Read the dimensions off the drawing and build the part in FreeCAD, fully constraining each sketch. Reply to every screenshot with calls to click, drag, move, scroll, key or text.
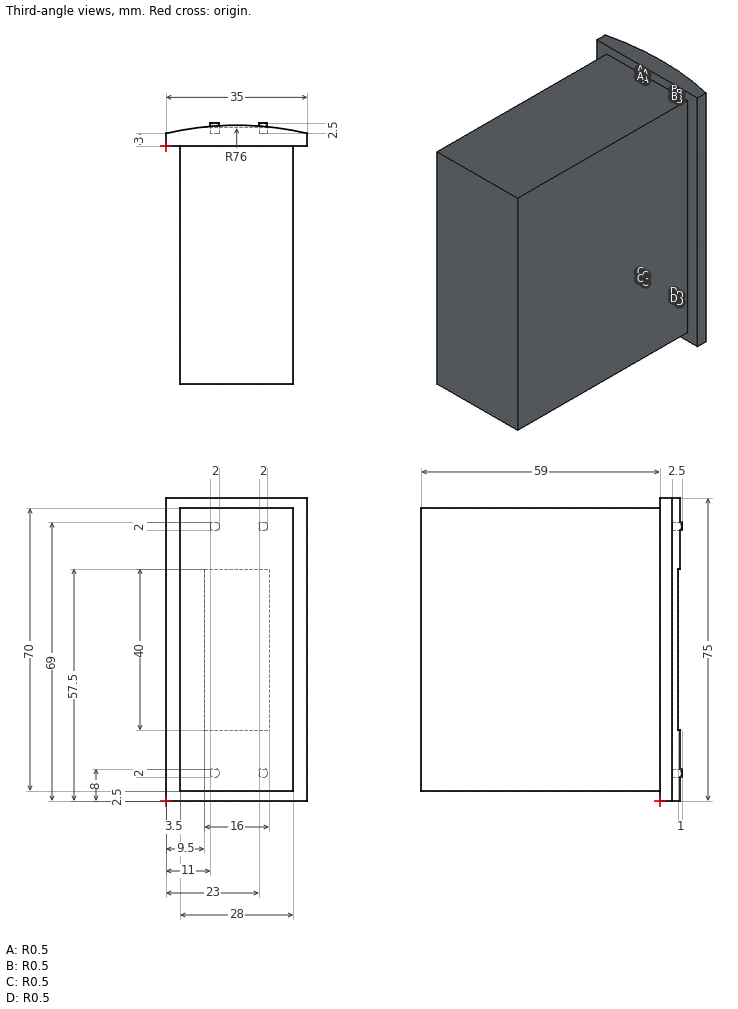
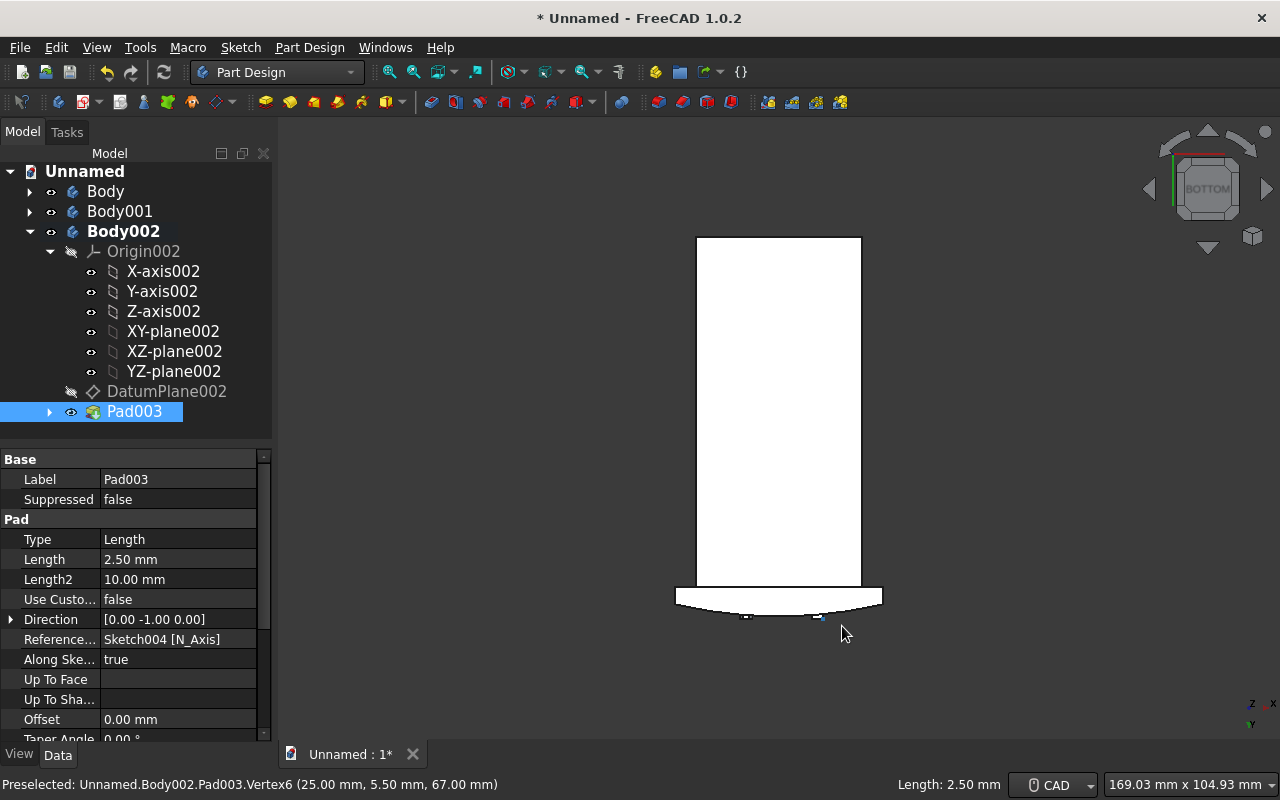
key(4)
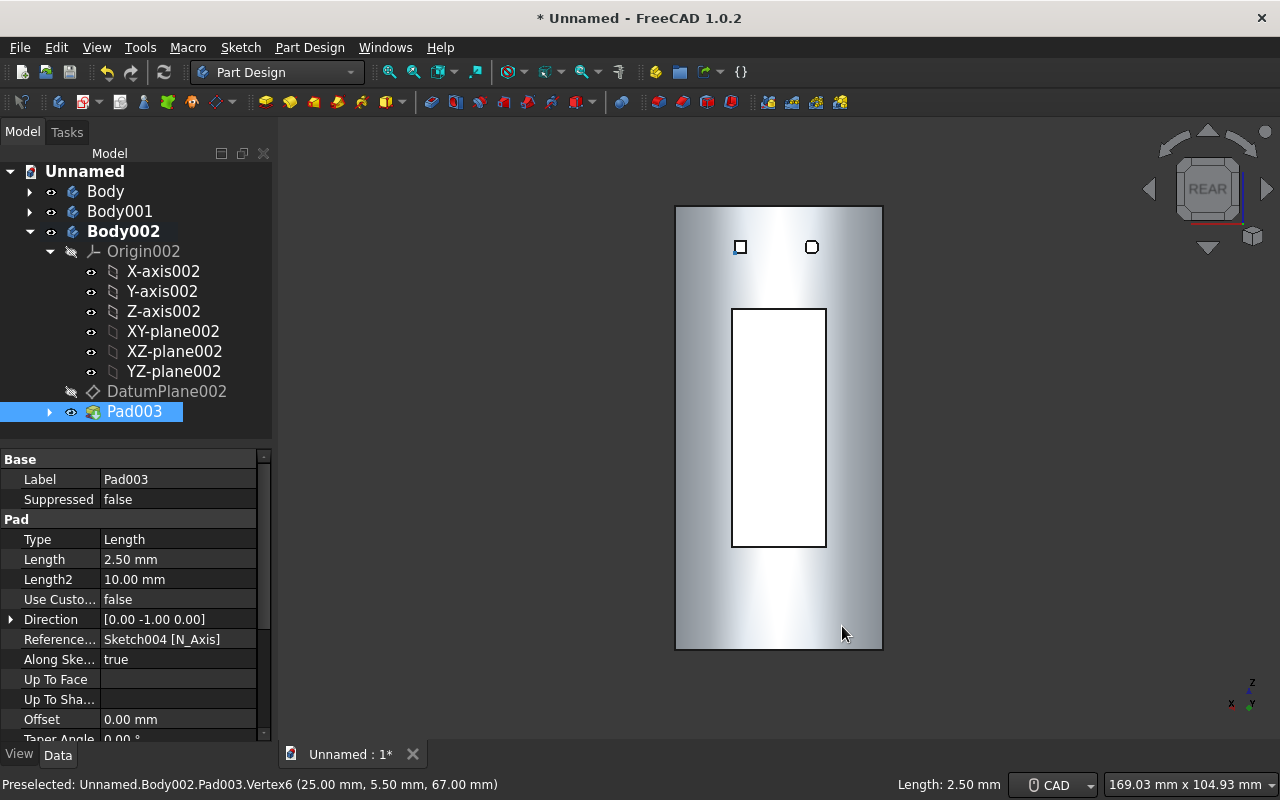
key(v)
key(f)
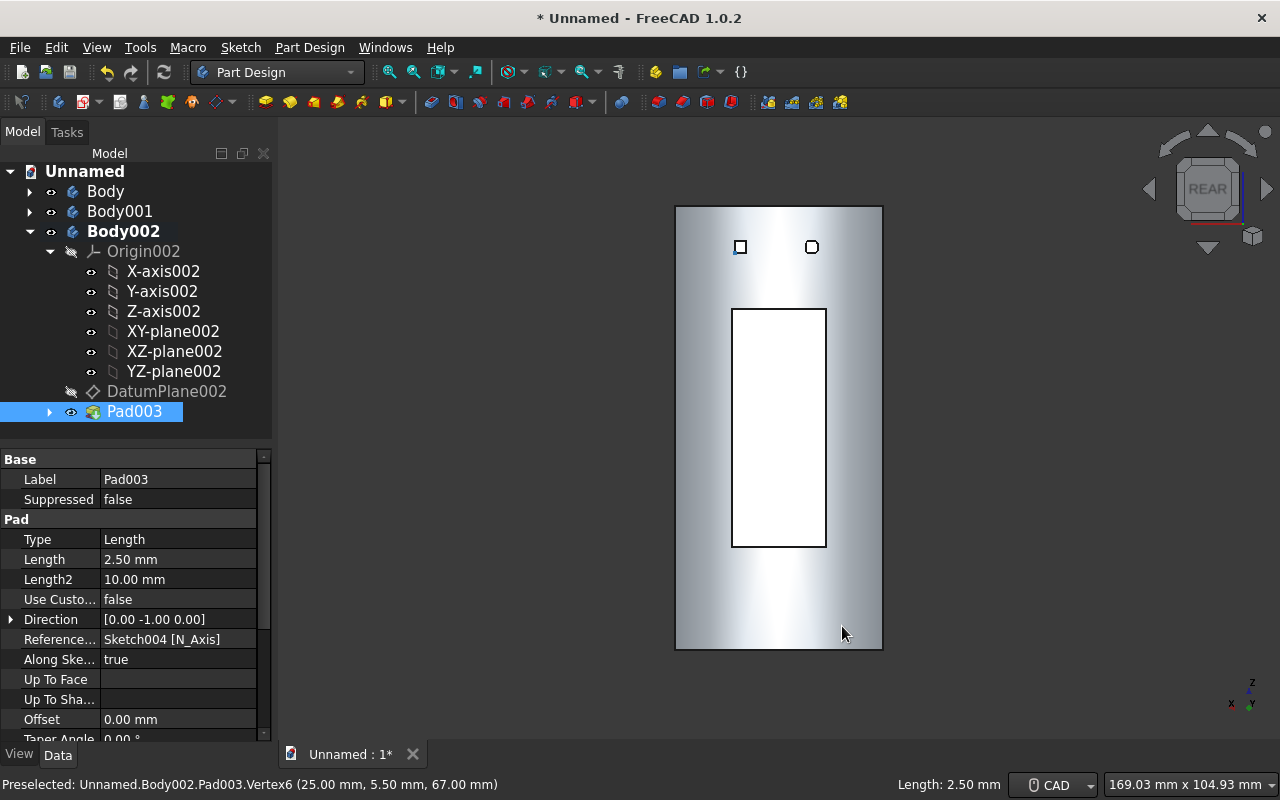
scroll(746, 240, up, 5)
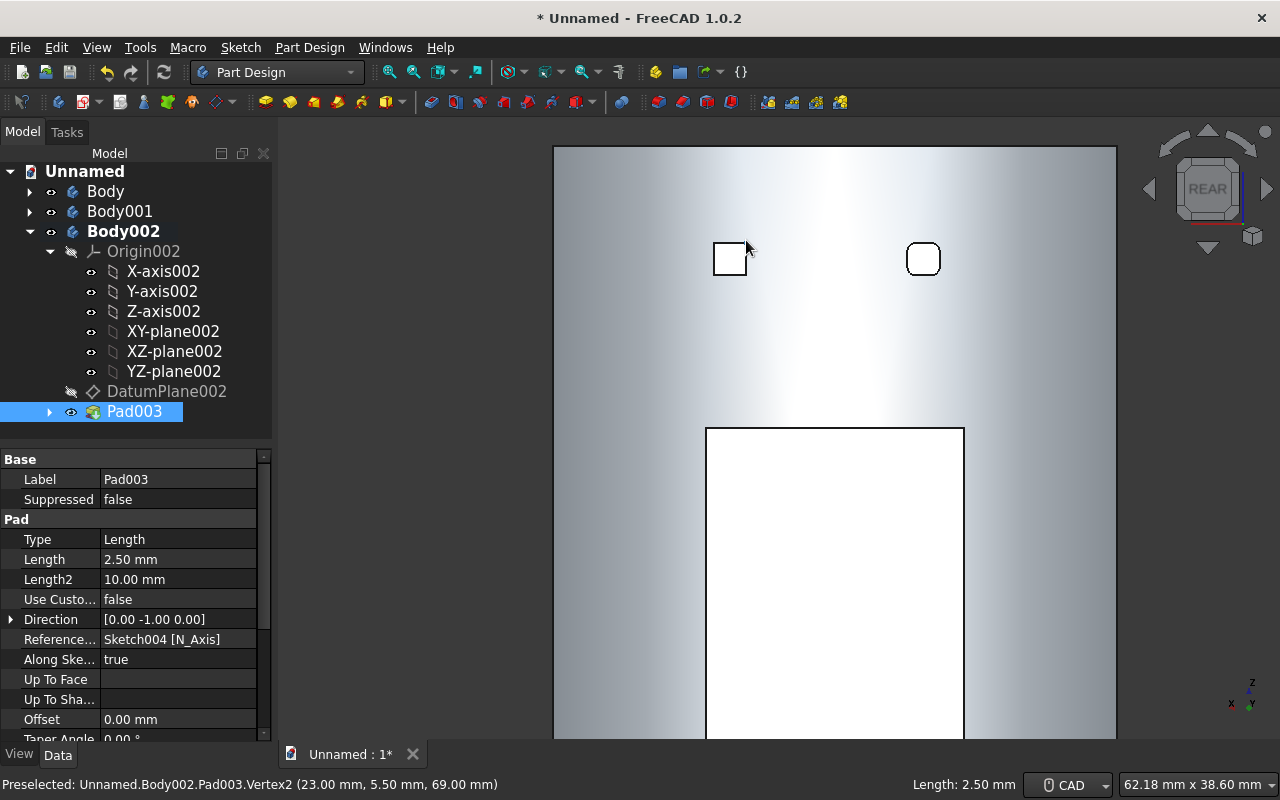
key(v)
key(f)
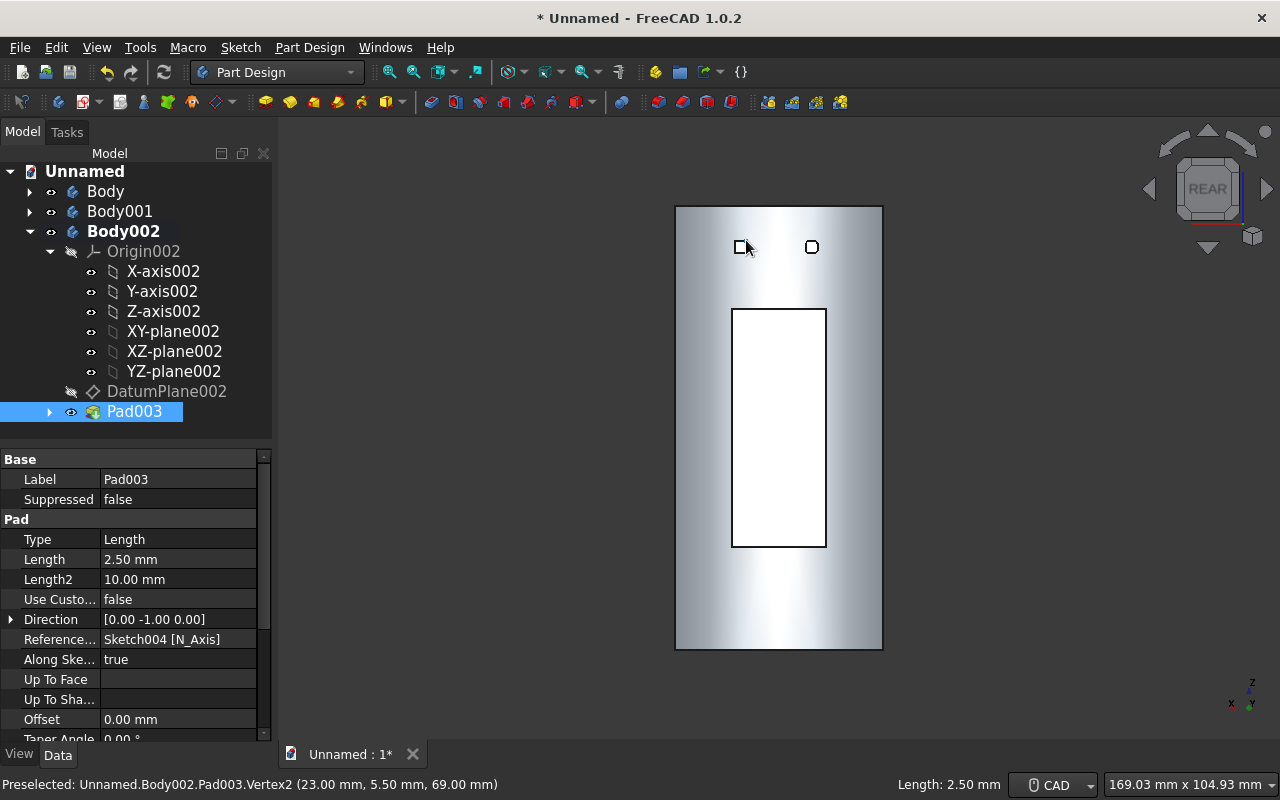
key(6)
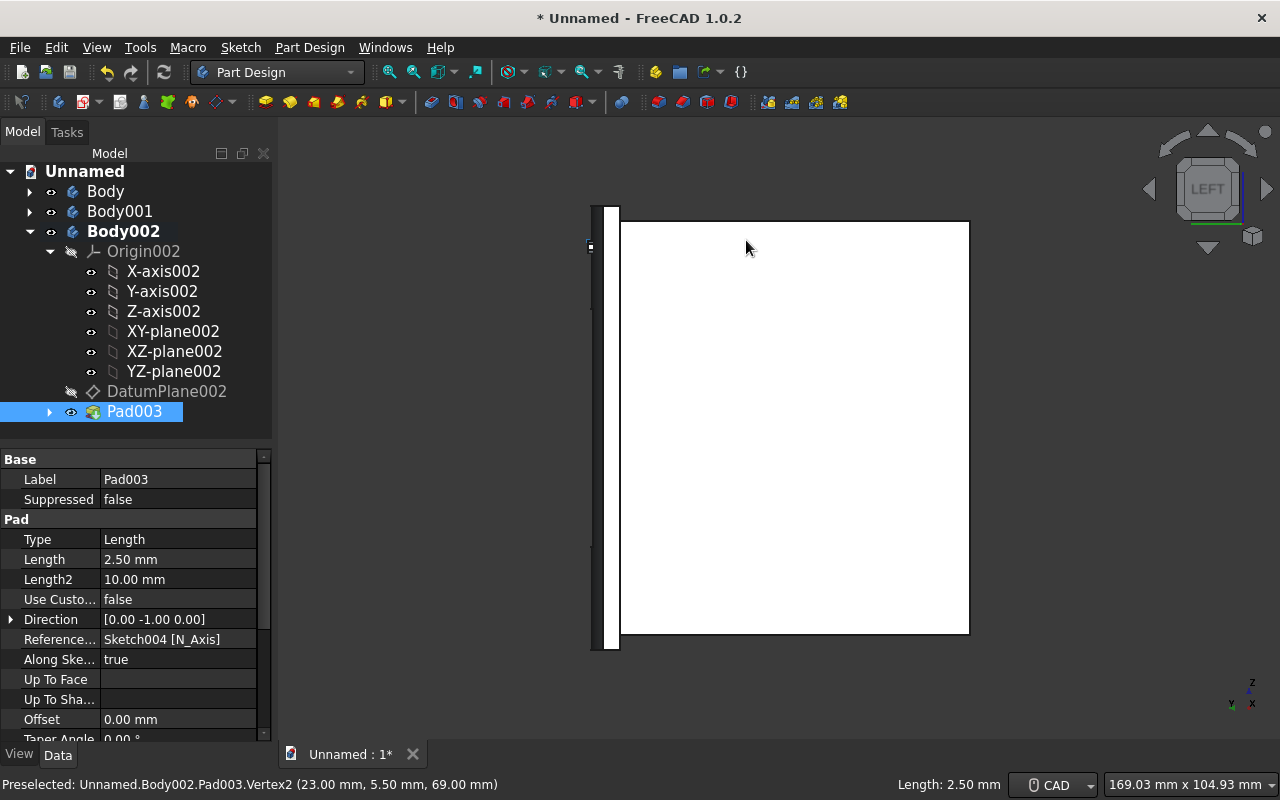
key(v)
key(f)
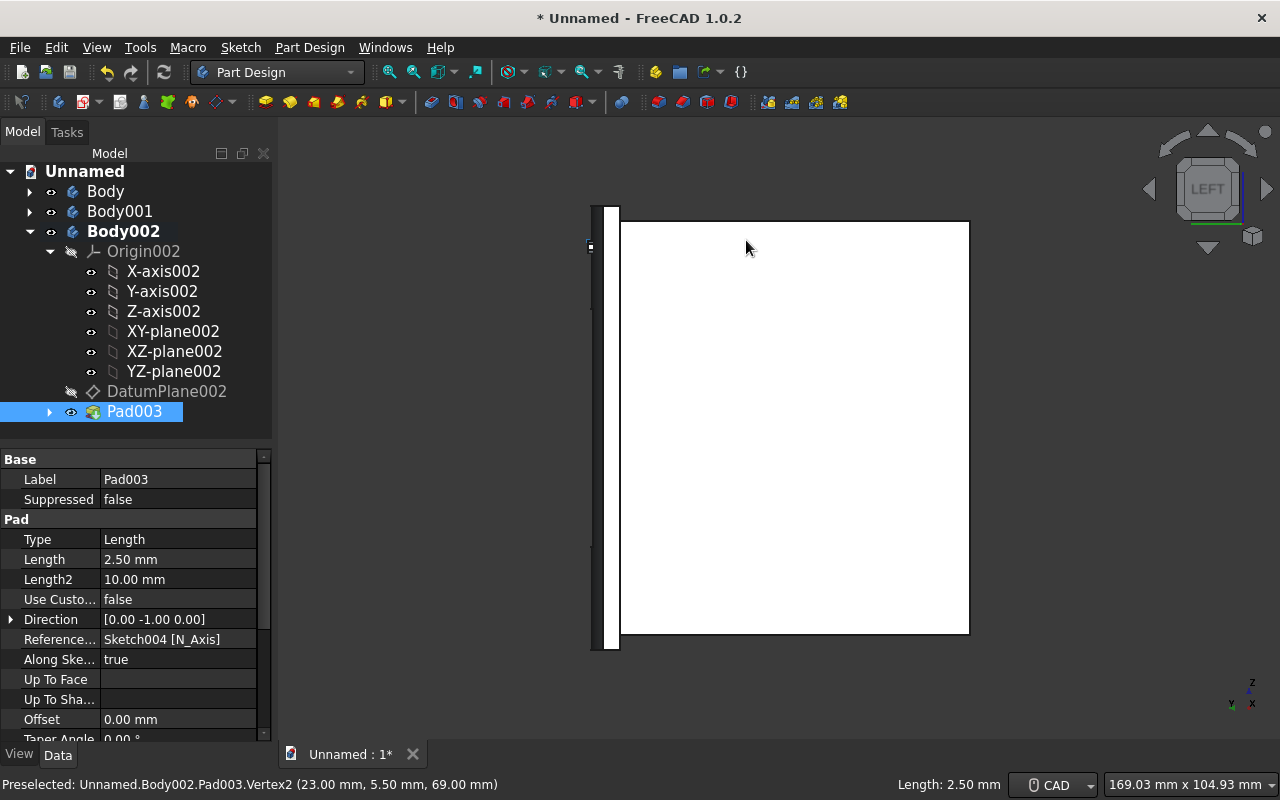
scroll(595, 240, up, 5)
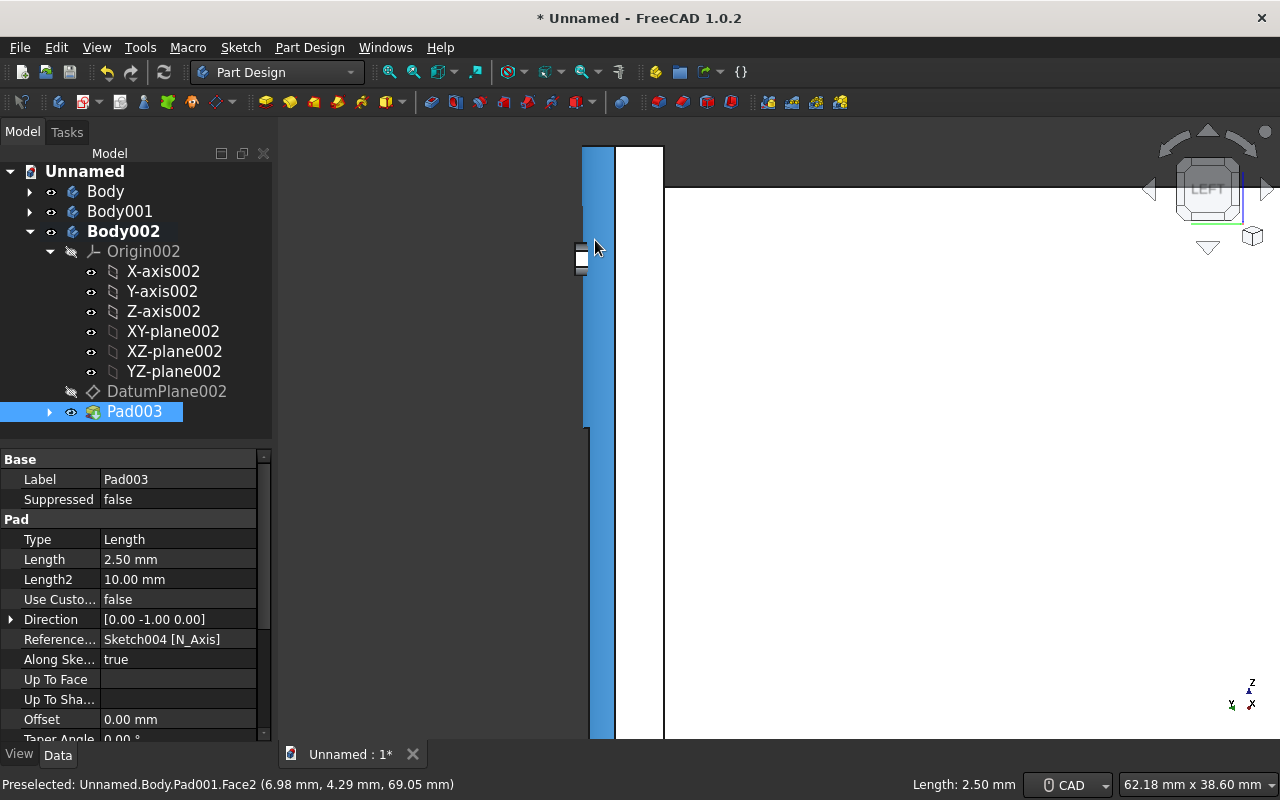
key(v)
key(f)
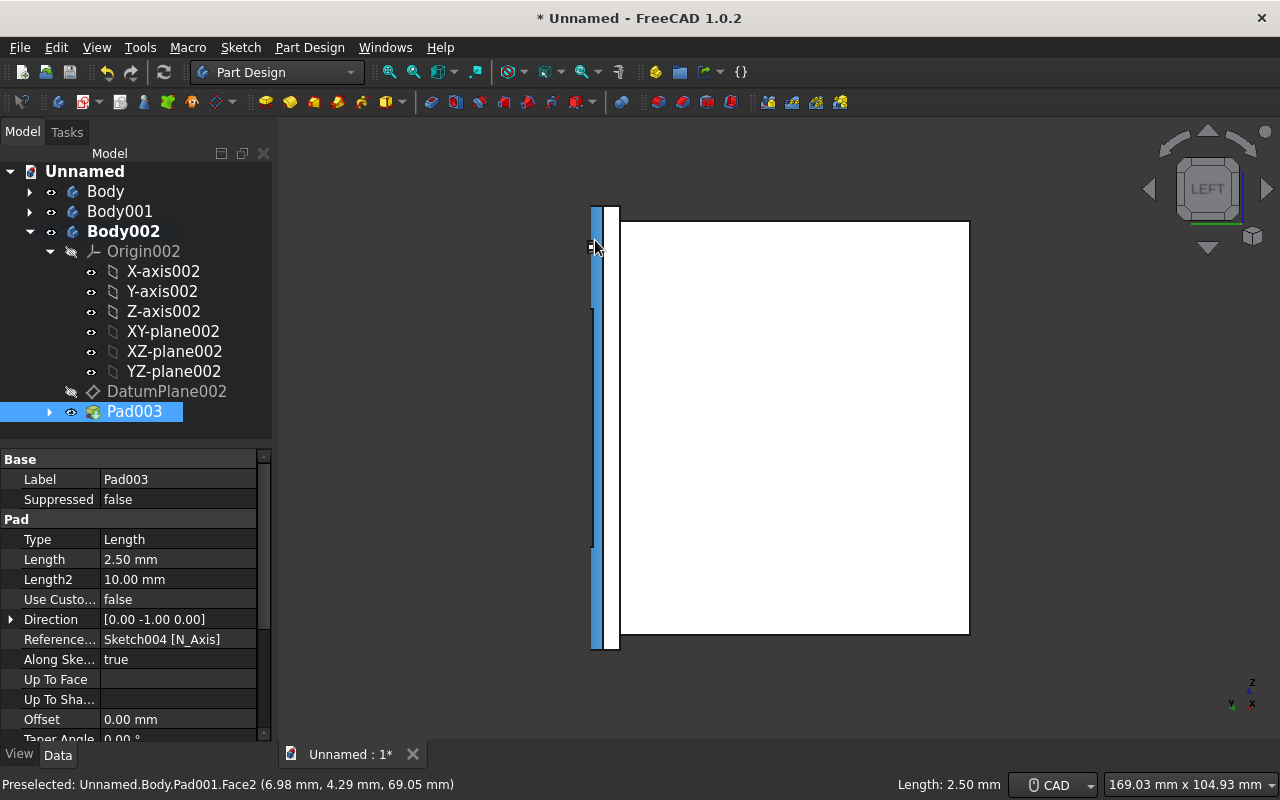
key(v)
key(3)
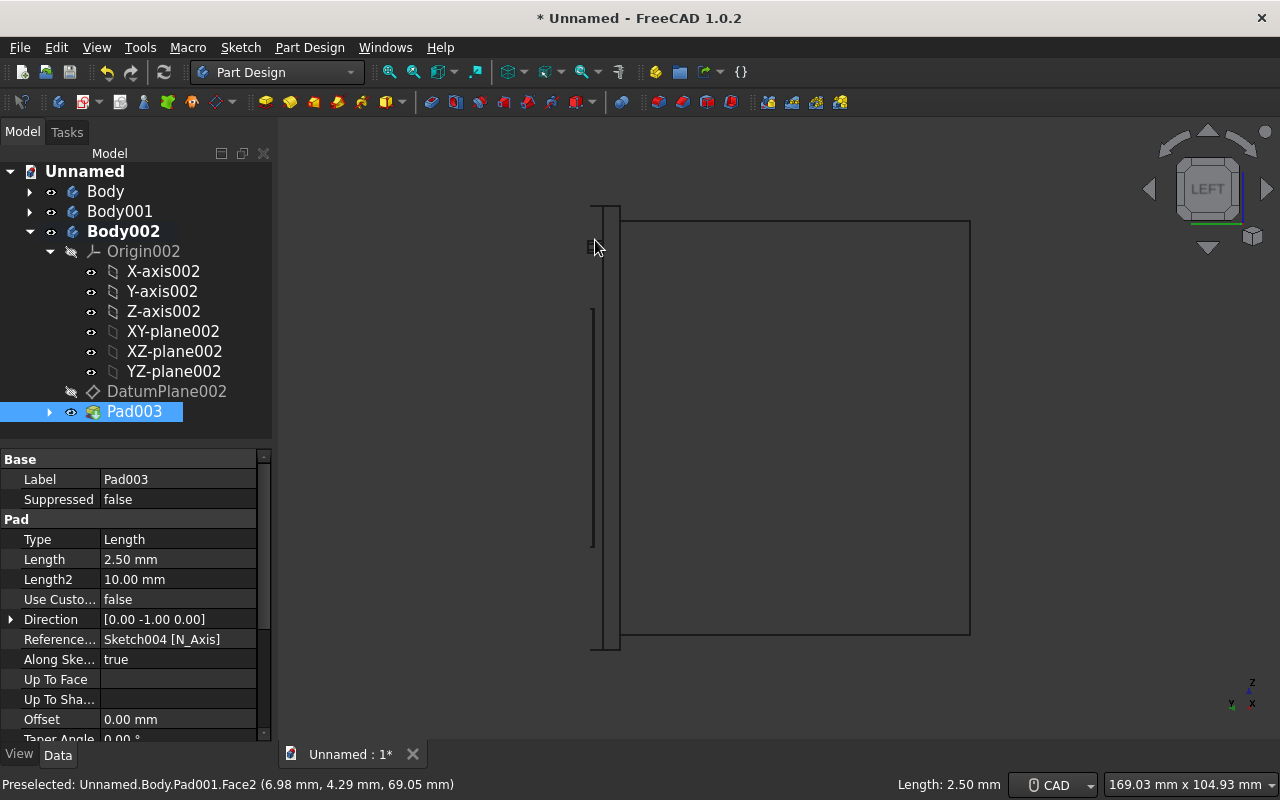
key(0)